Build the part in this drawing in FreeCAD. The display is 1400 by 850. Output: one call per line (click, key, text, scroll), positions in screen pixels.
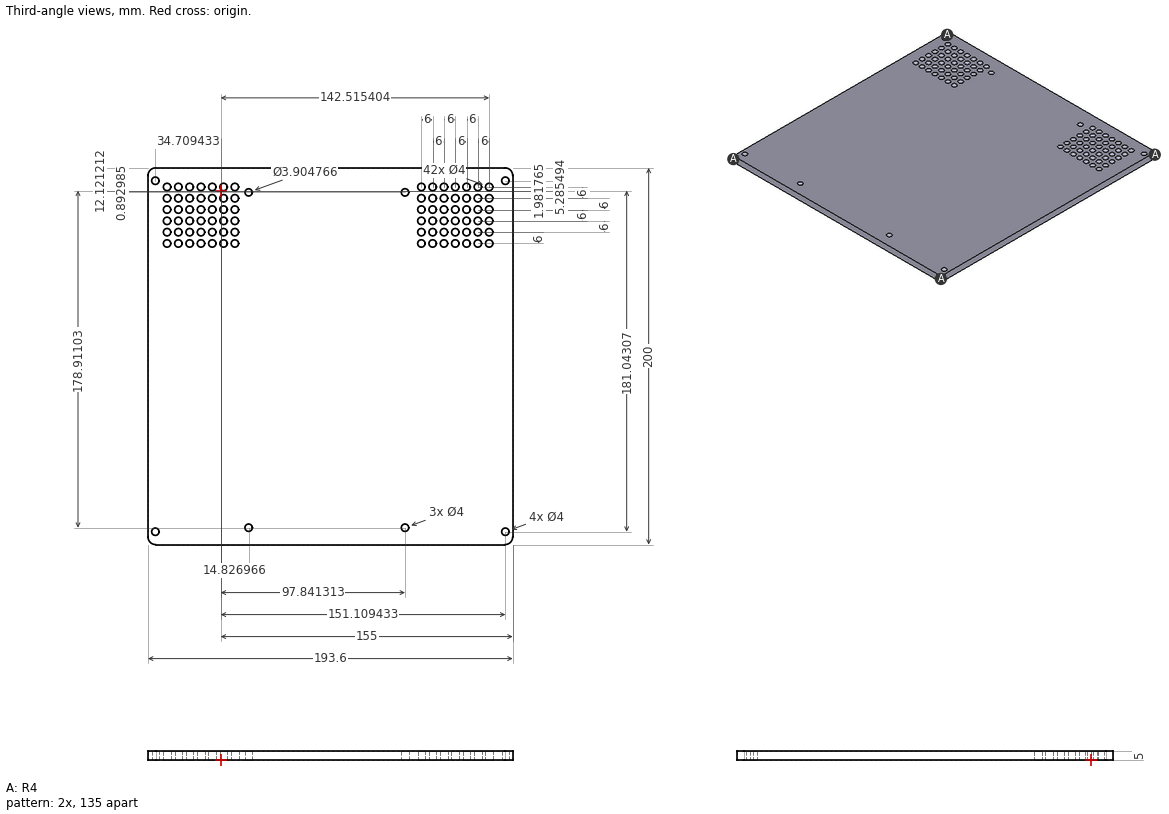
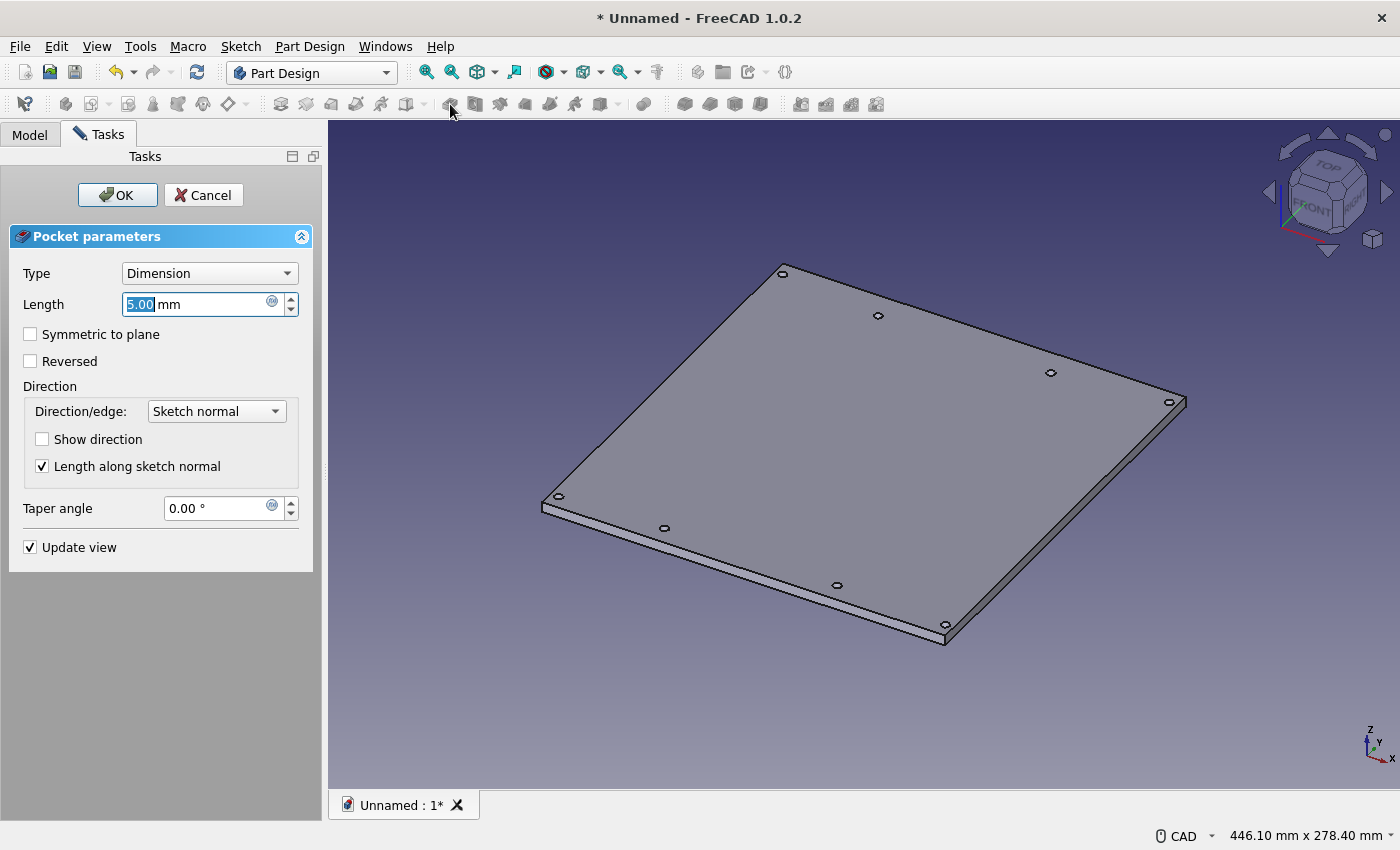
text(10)
key(Tab)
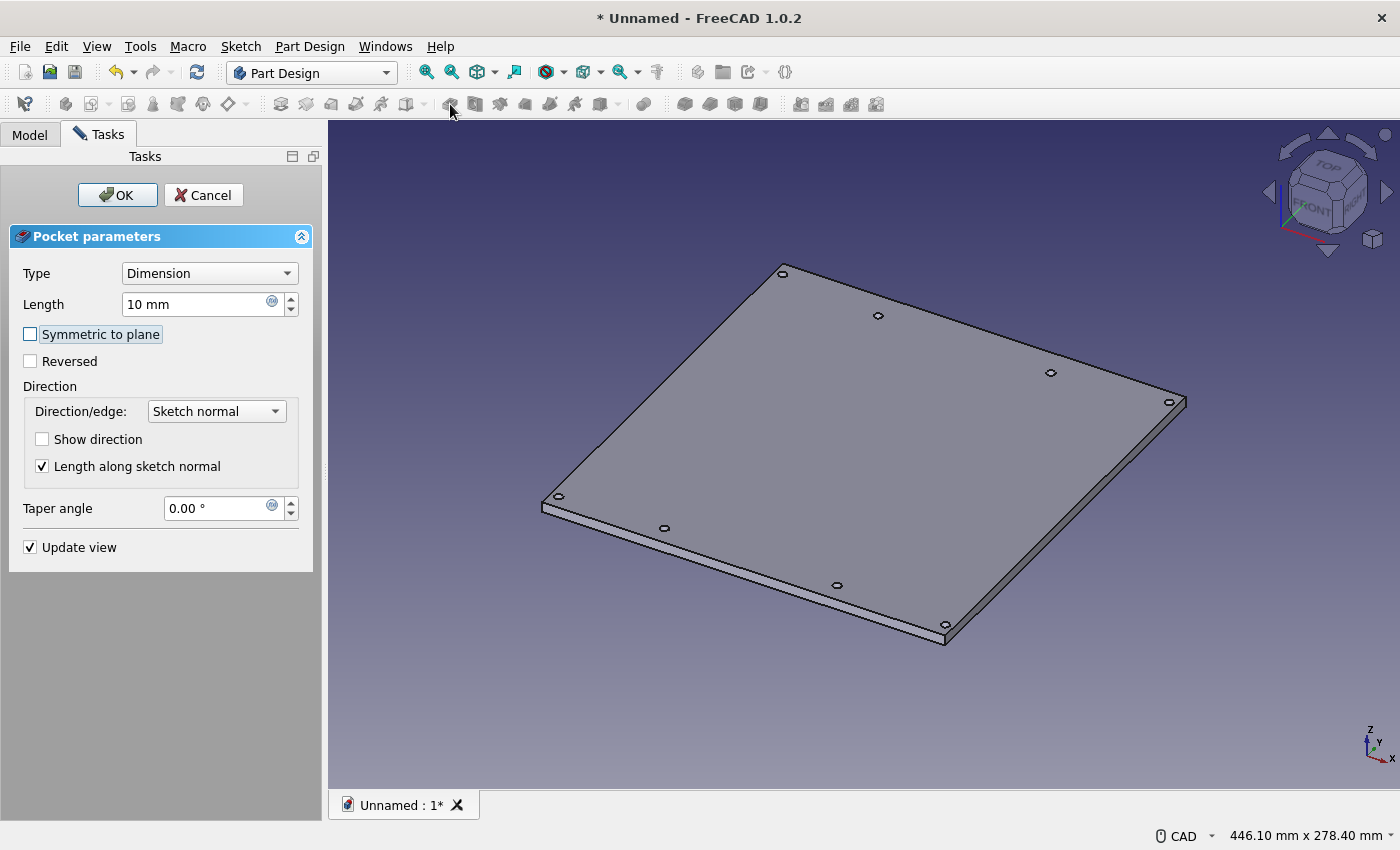
click(118, 195)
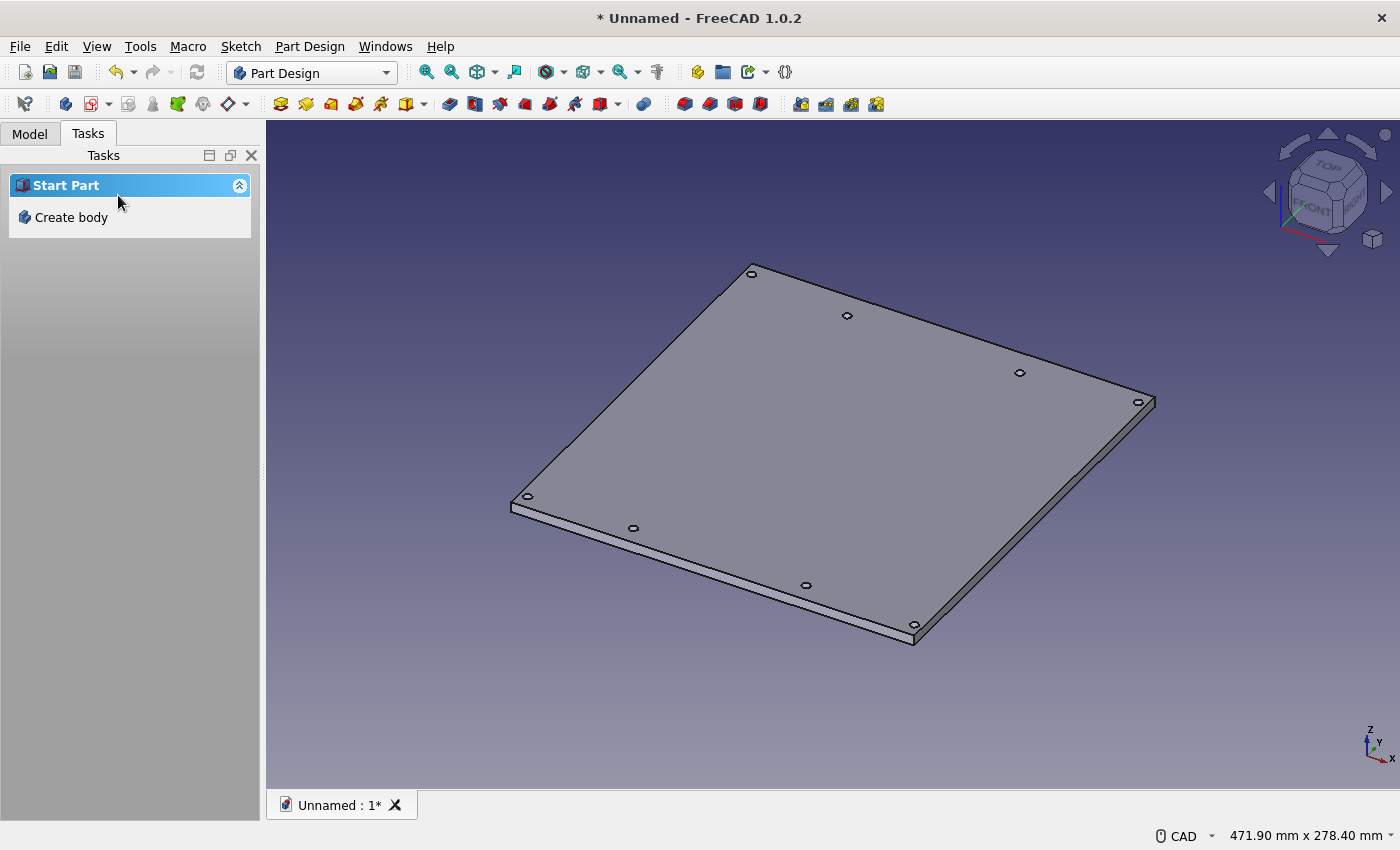
click(914, 641)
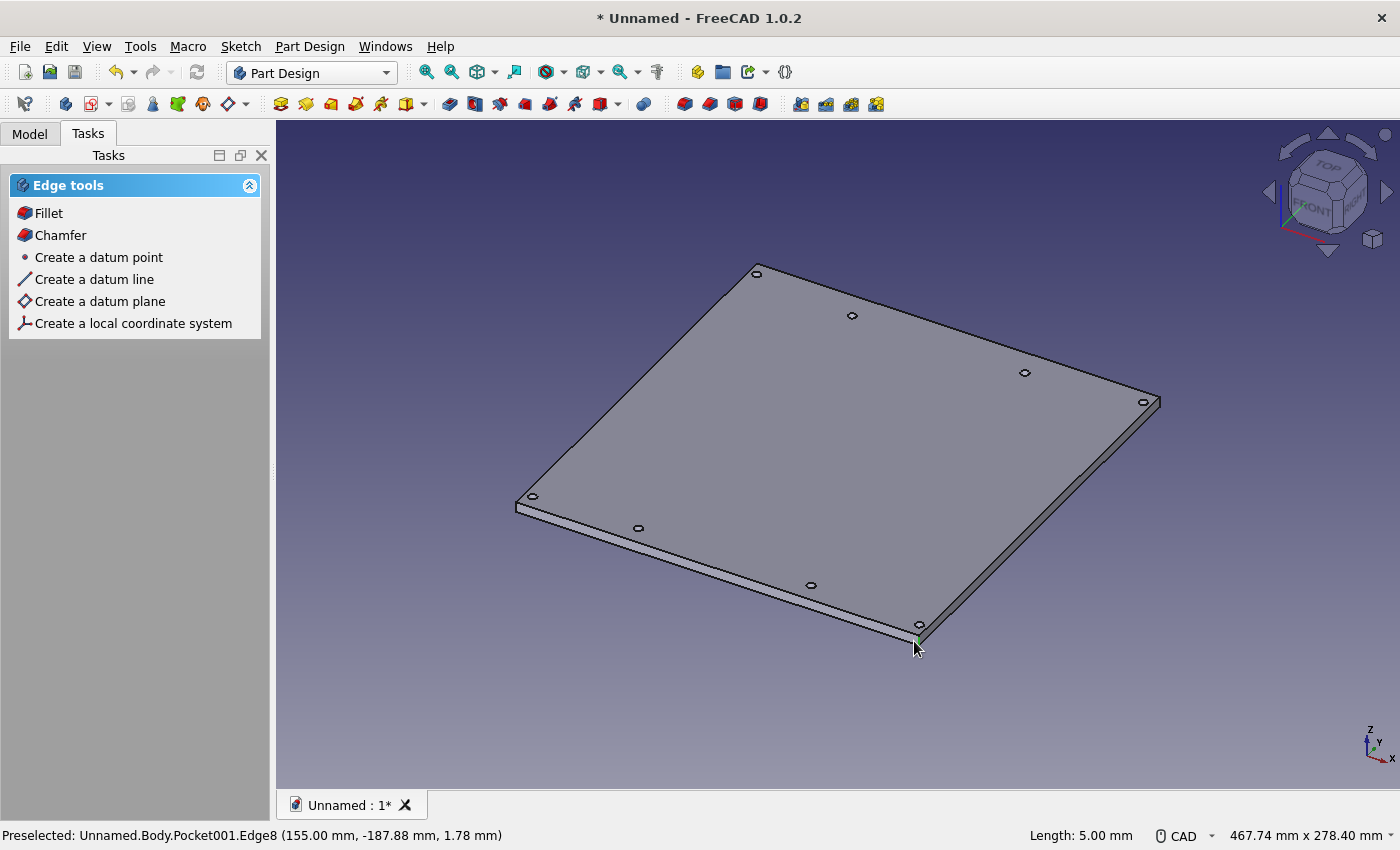
scroll(757, 267, up, 7)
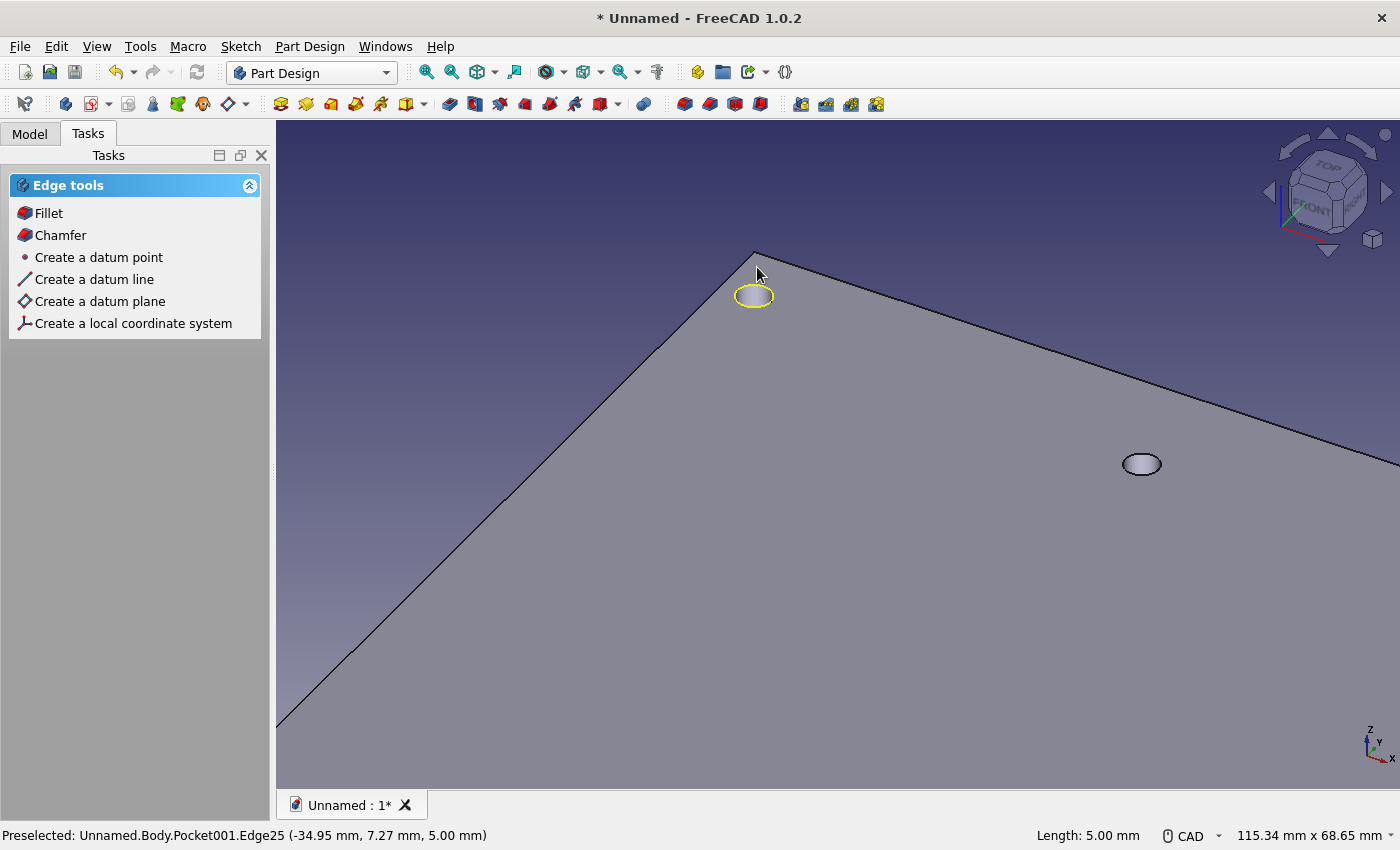
click(427, 72)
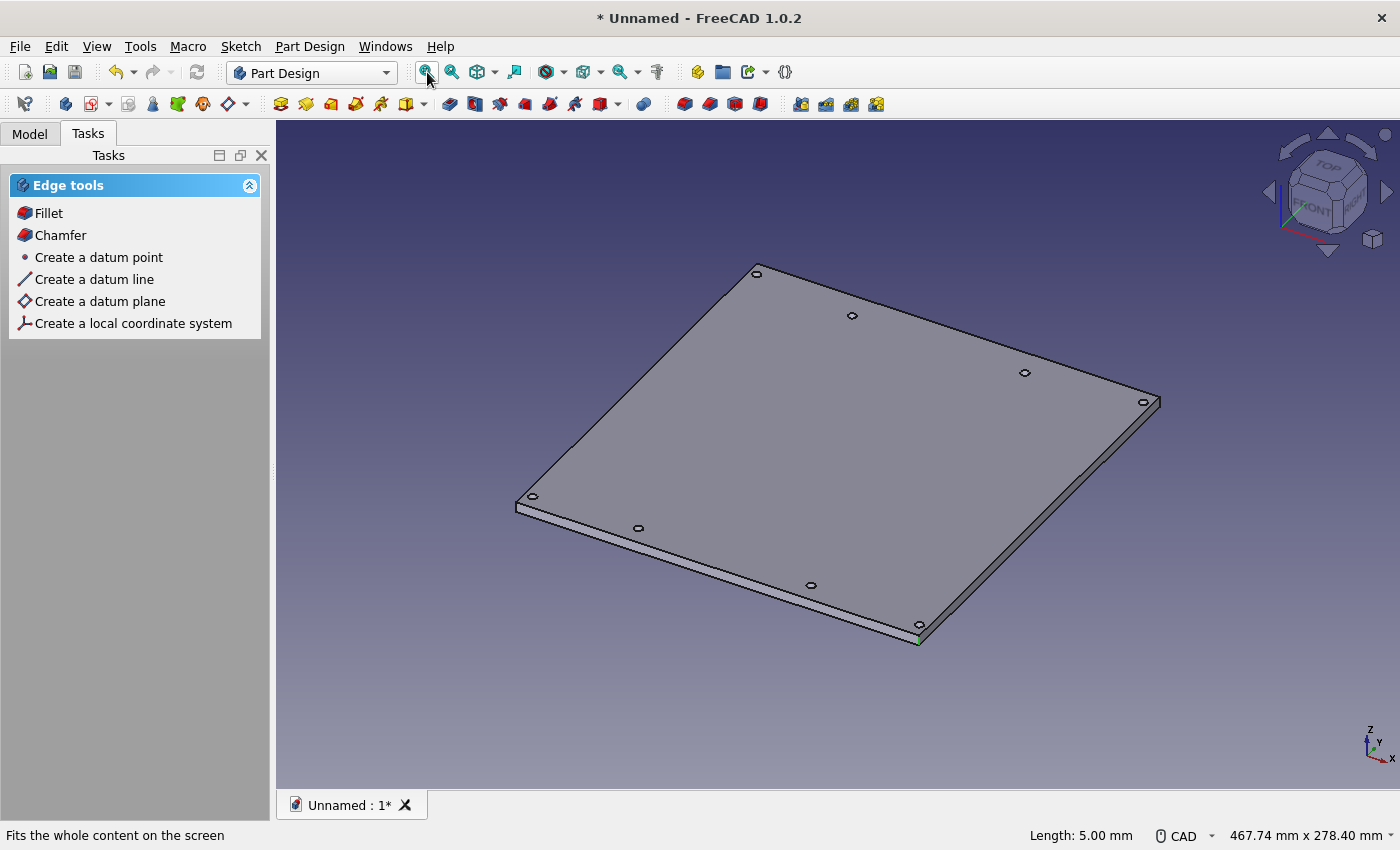
key(0)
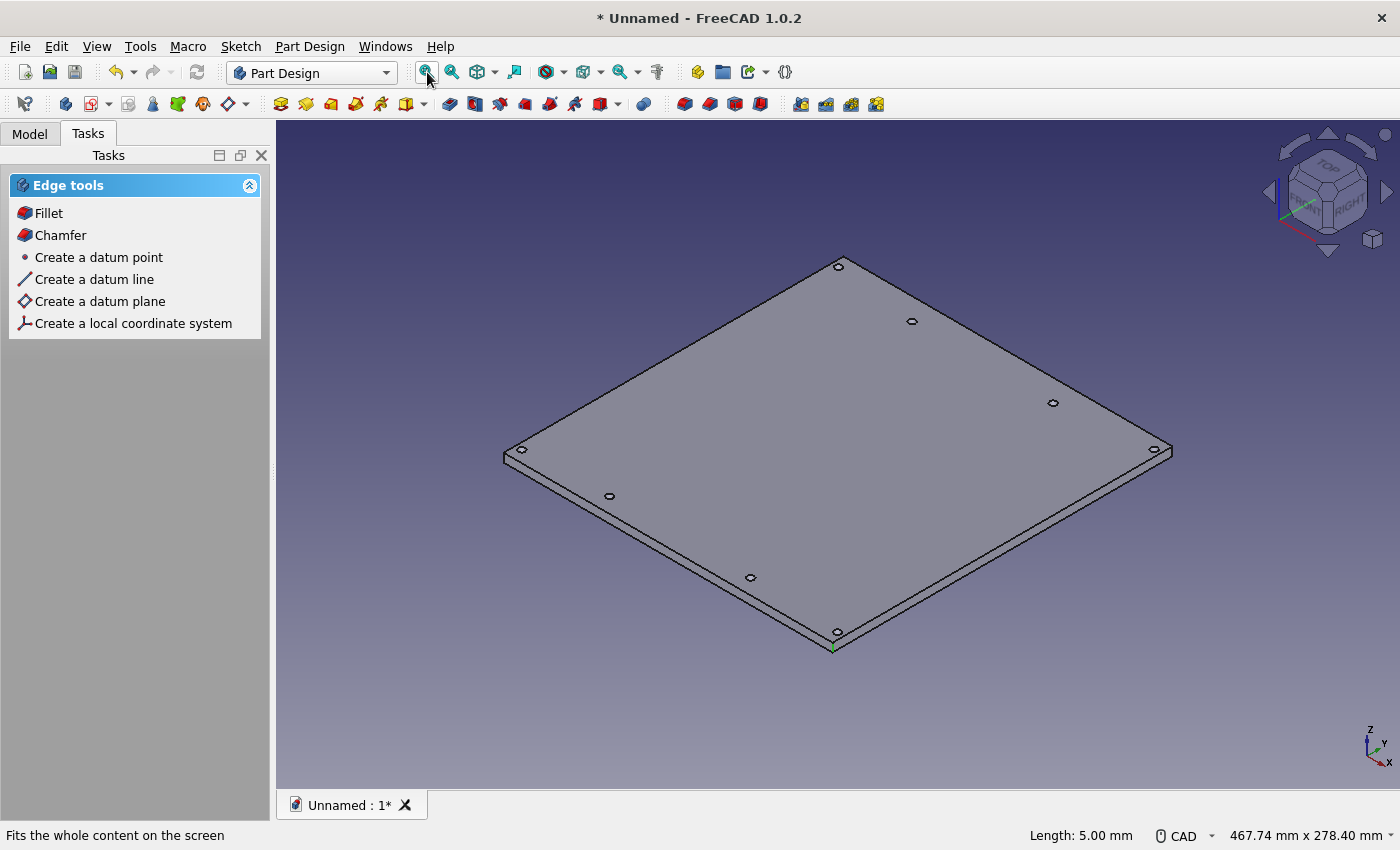
scroll(843, 260, up, 7)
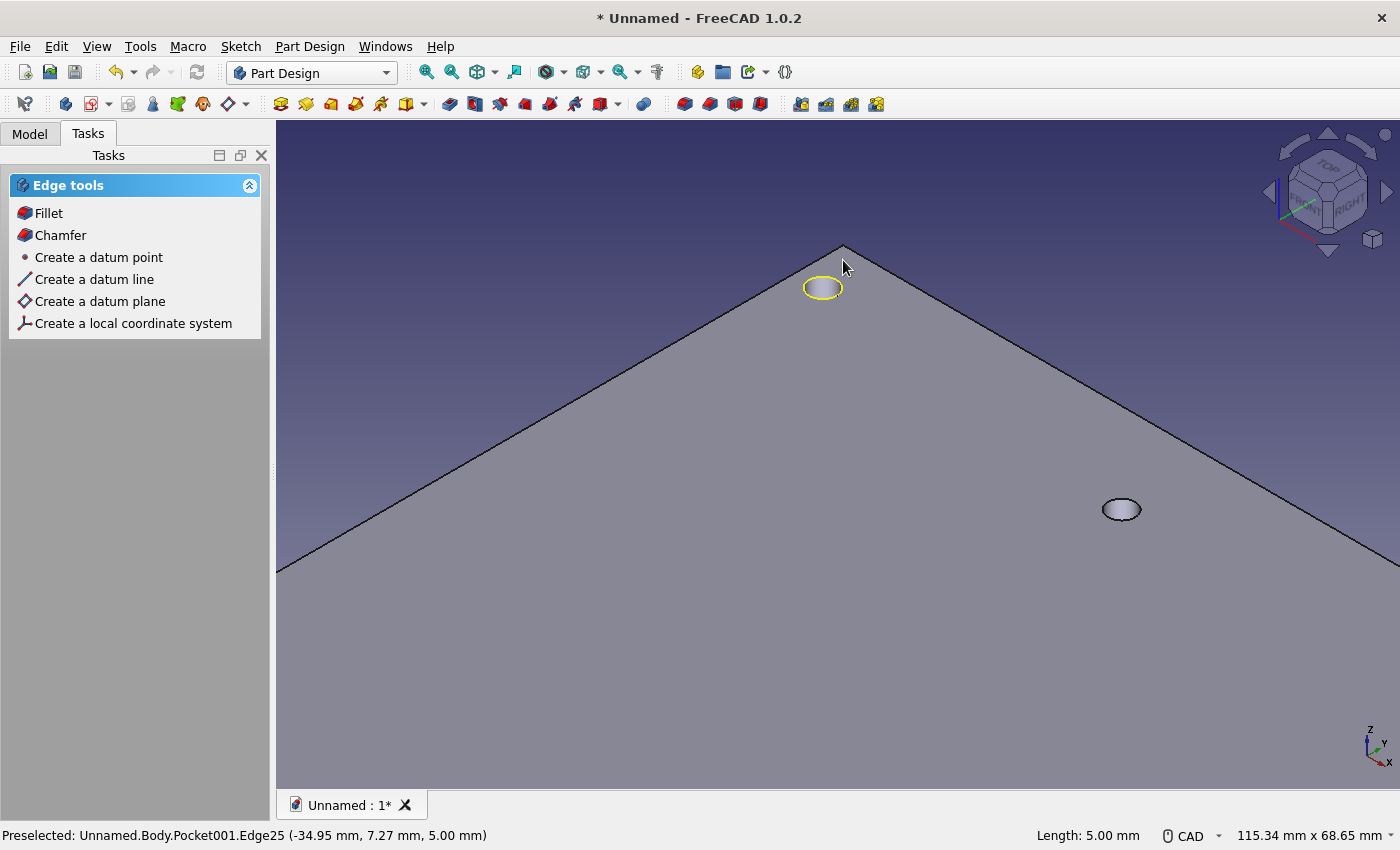
click(427, 72)